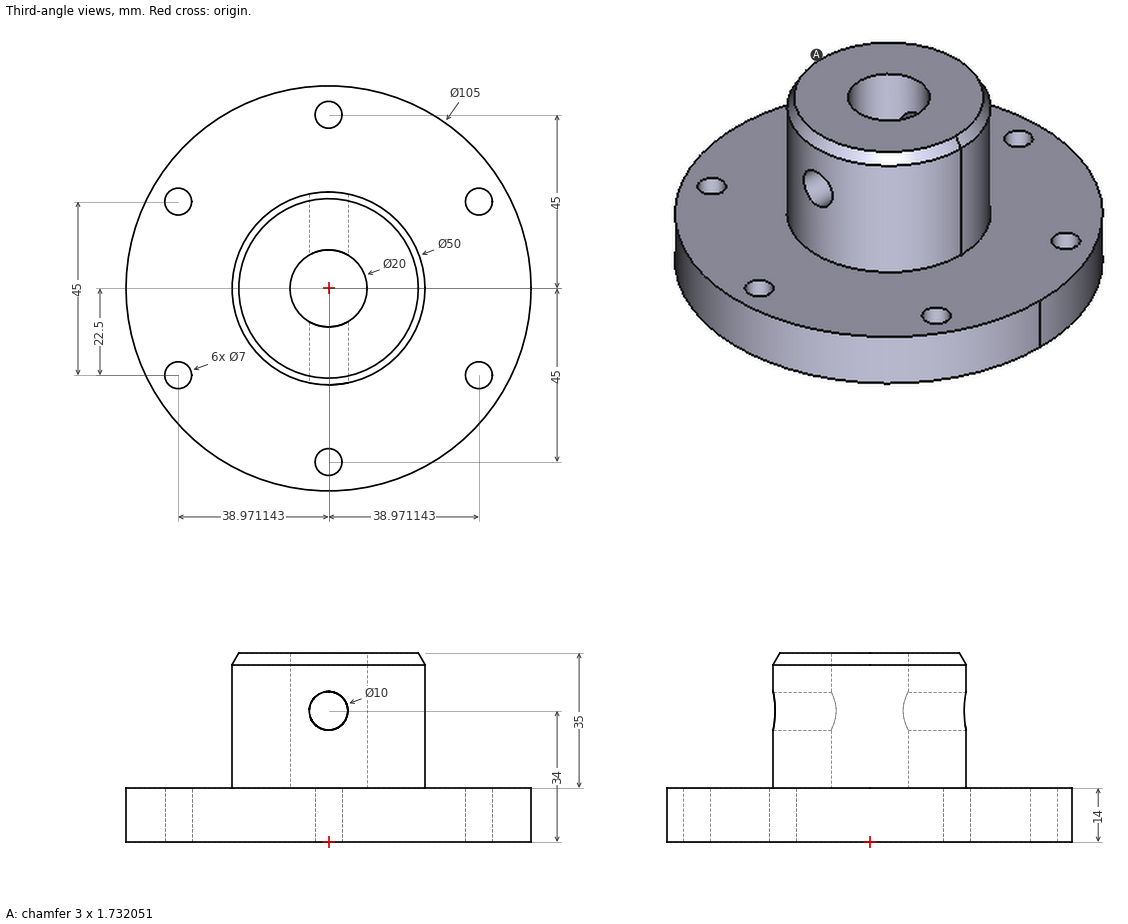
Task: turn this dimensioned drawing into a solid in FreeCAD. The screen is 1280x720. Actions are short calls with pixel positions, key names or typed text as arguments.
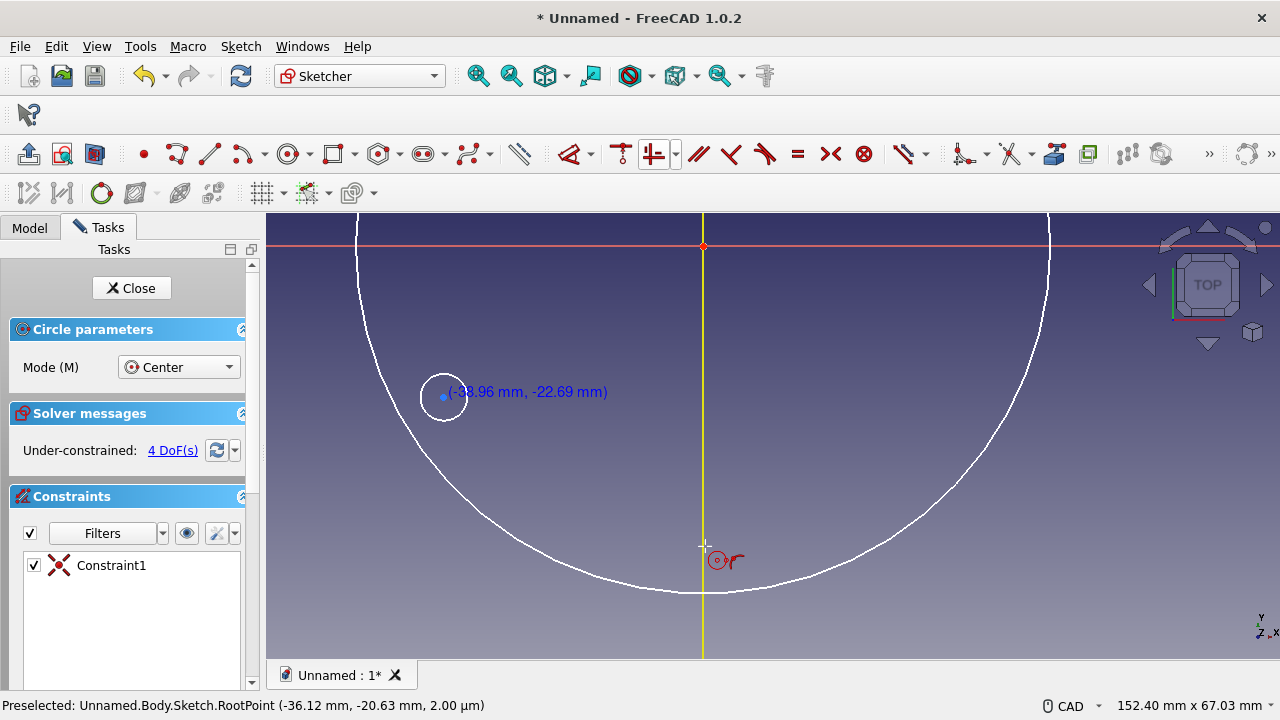
click(703, 546)
click(720, 529)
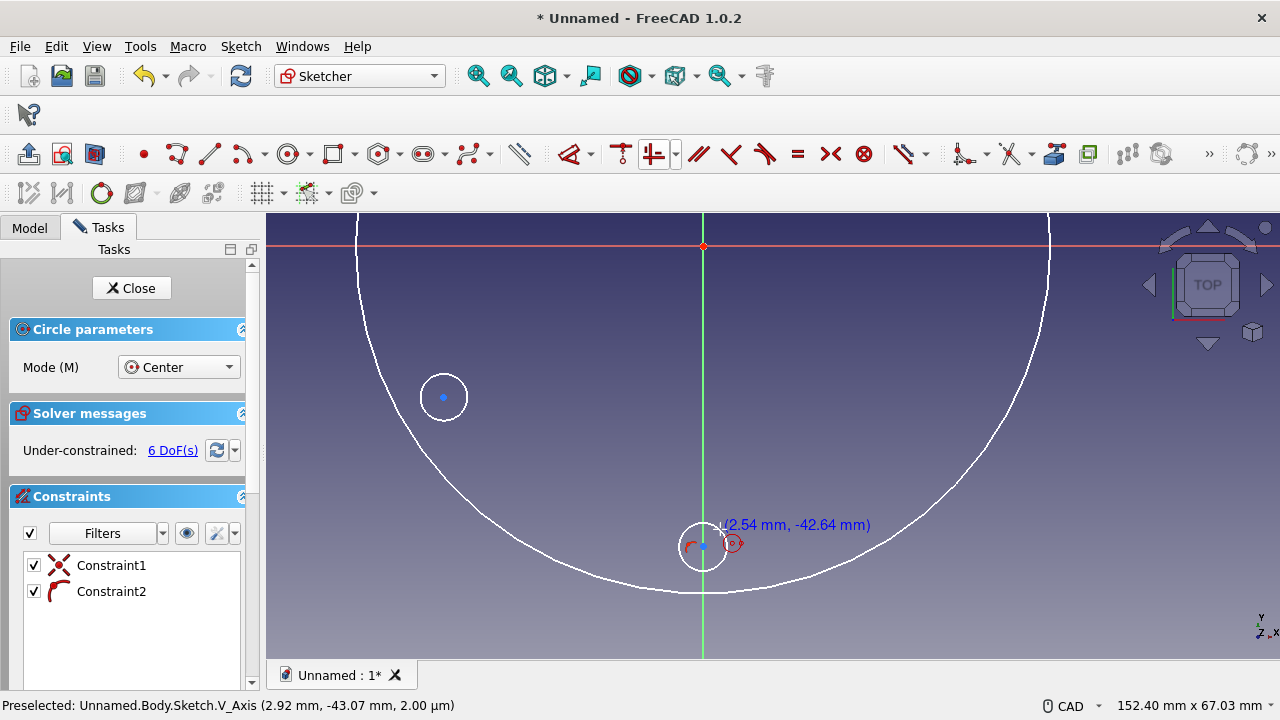
click(962, 396)
click(979, 380)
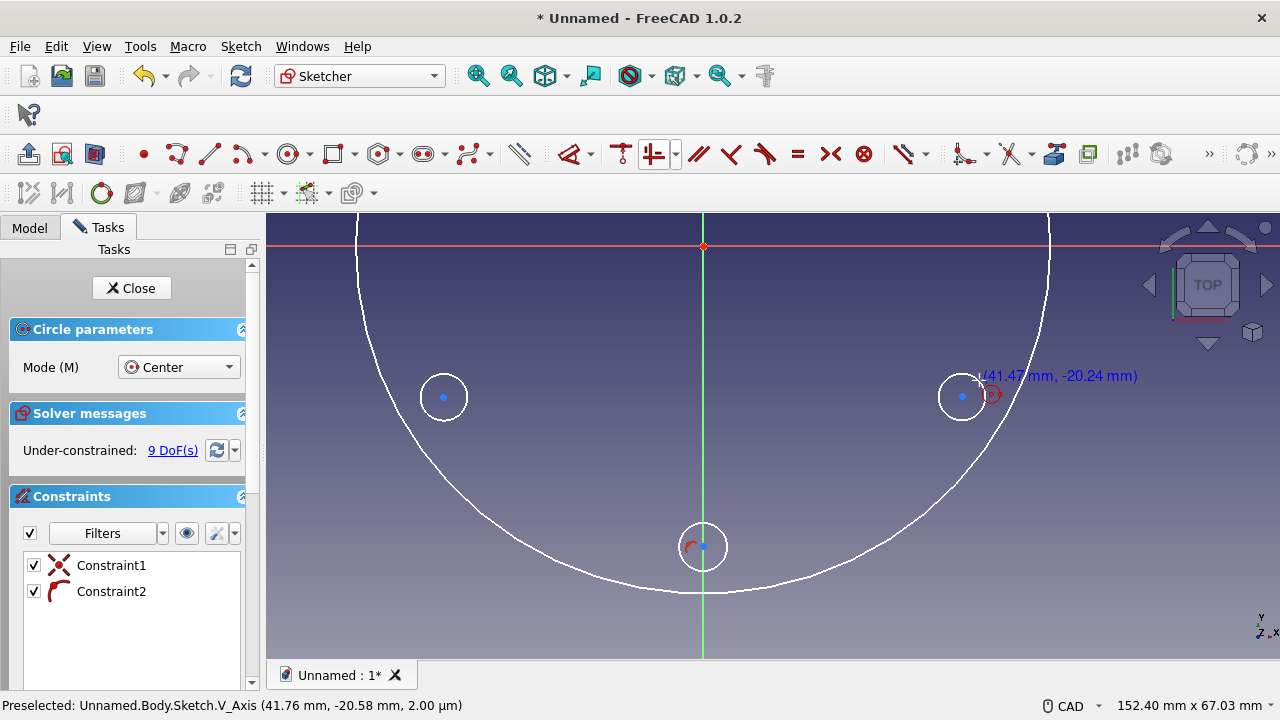
scroll(705, 546, down, 5)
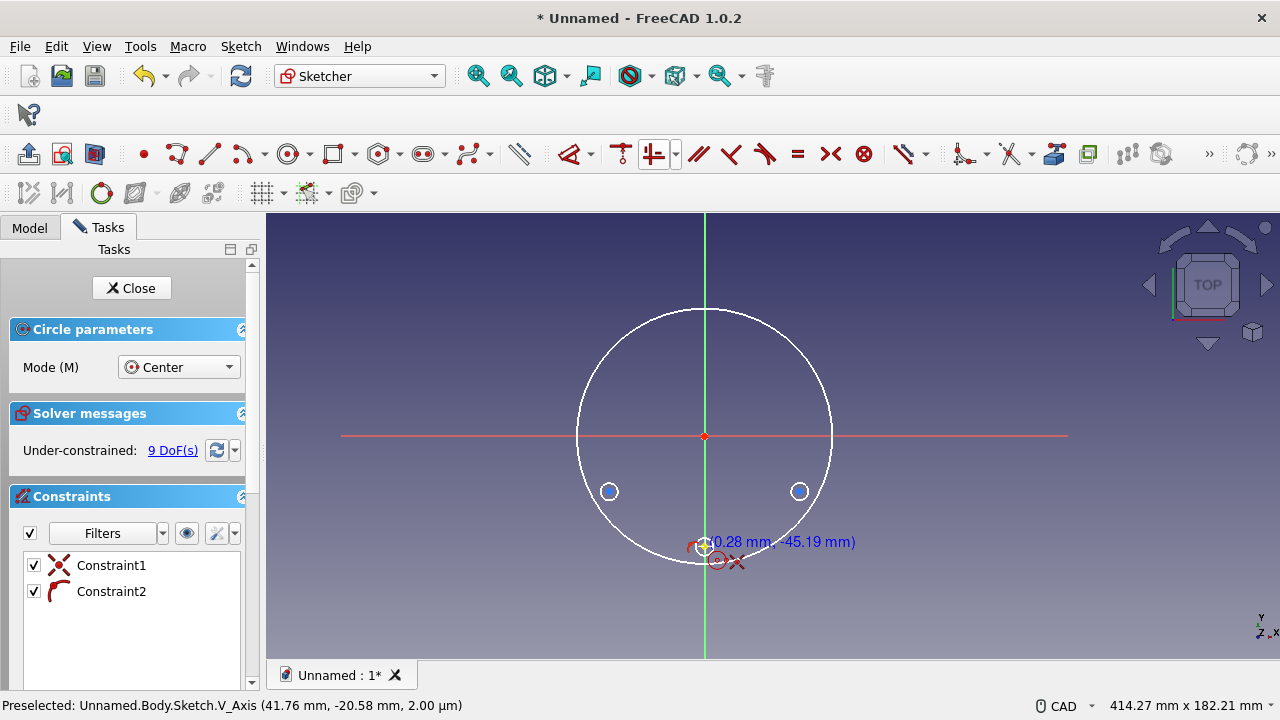
scroll(609, 381, up, 5)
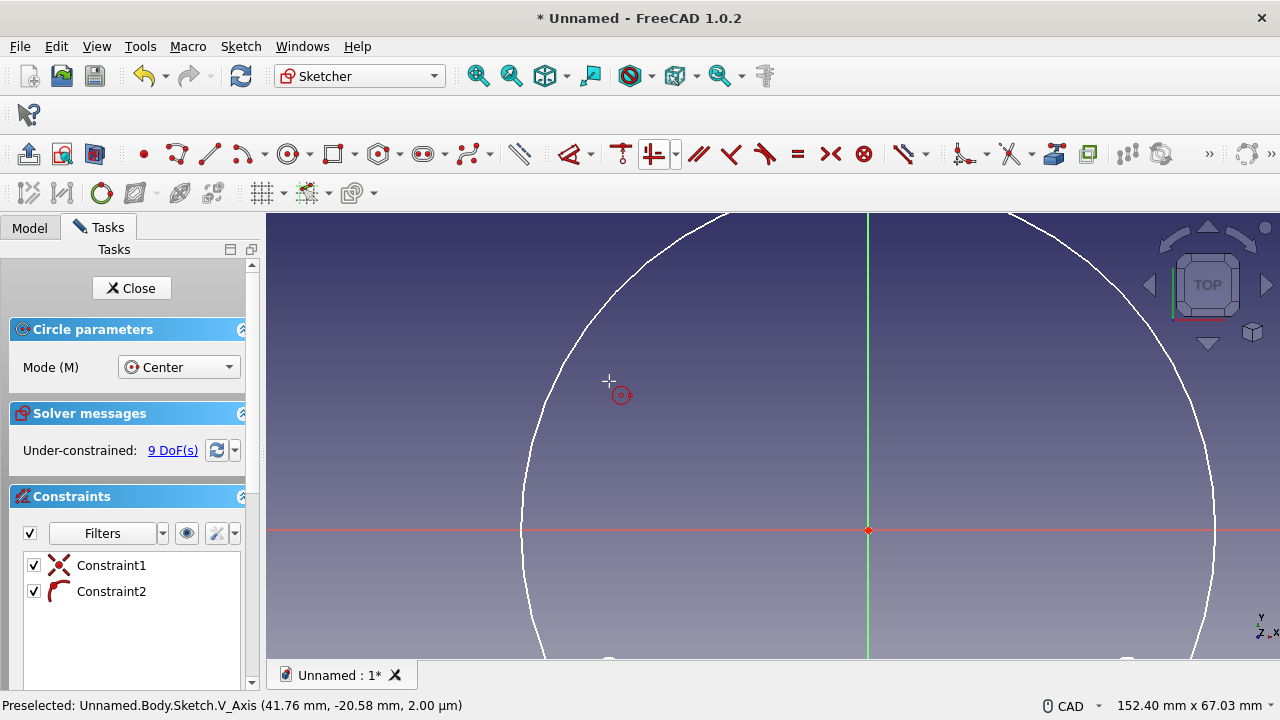
click(609, 381)
click(625, 364)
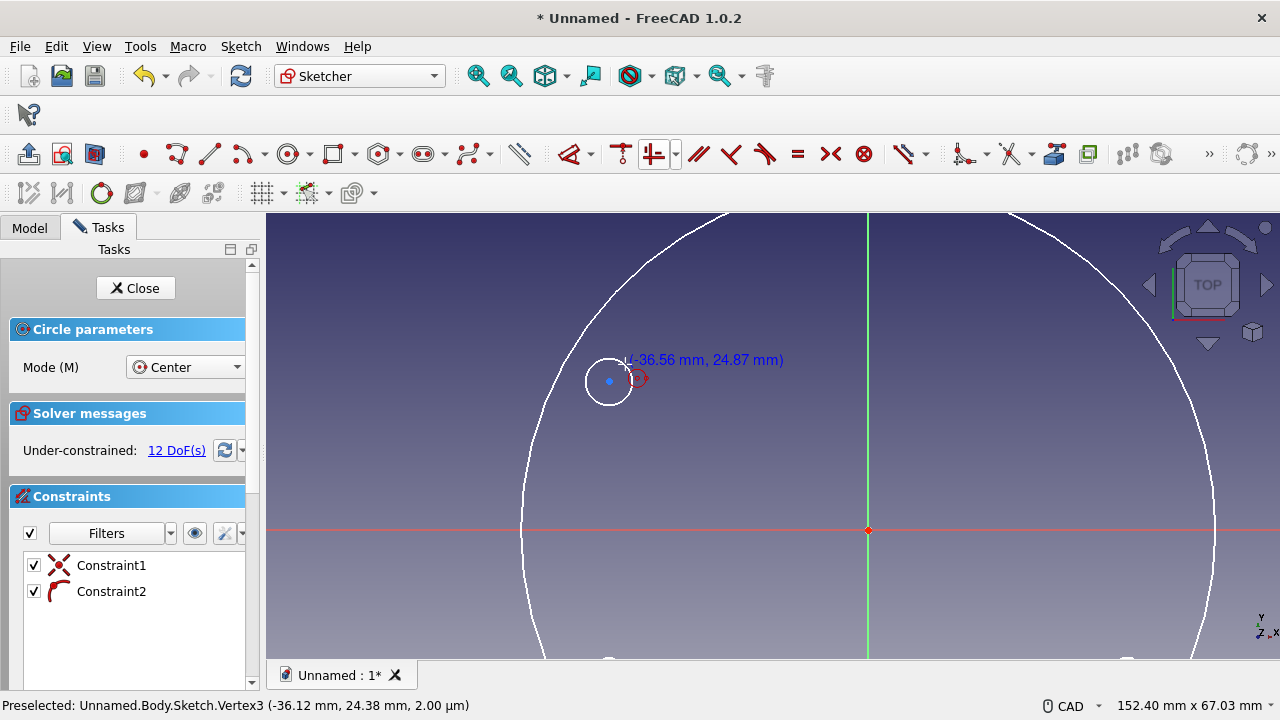
scroll(609, 381, down, 5)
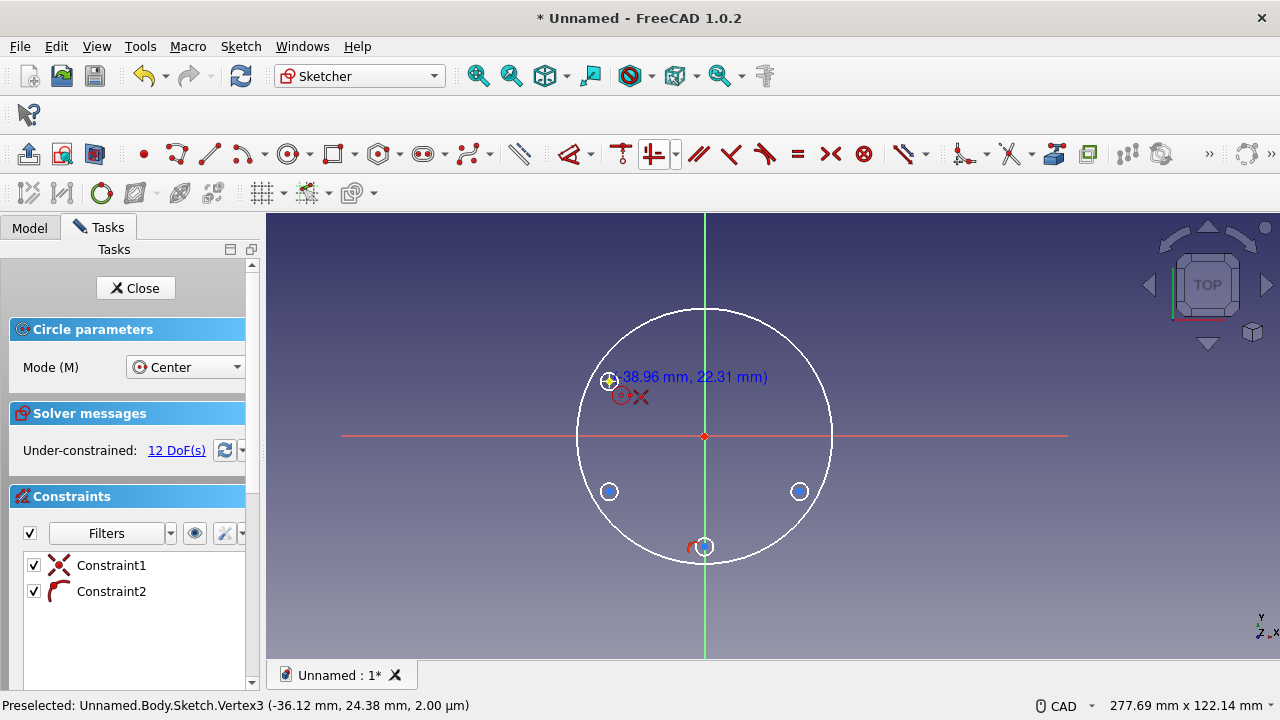
scroll(800, 381, up, 5)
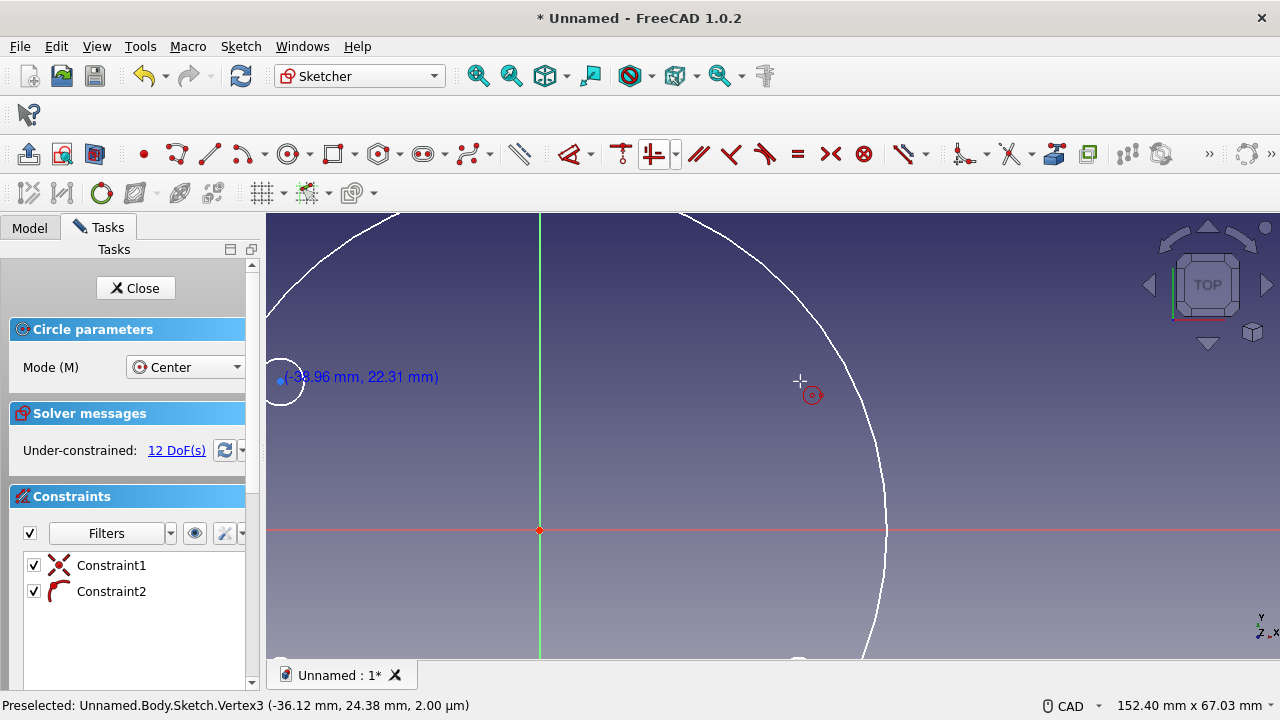
click(799, 381)
click(815, 364)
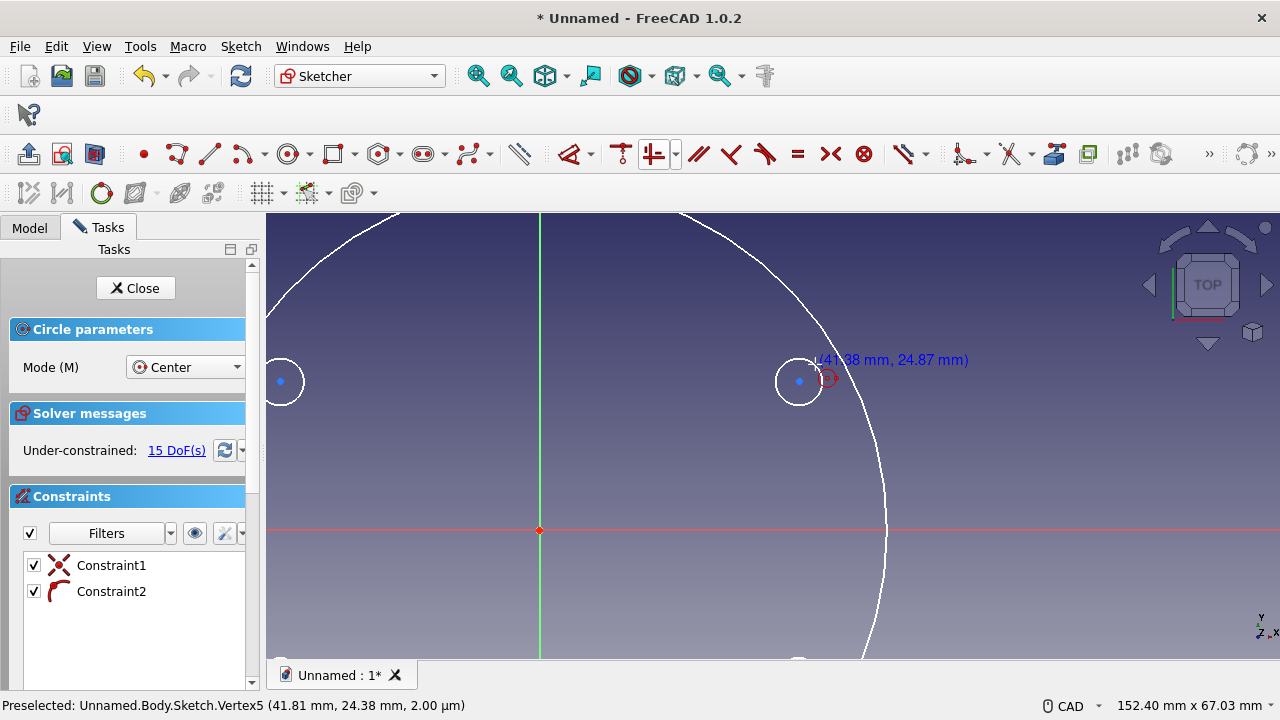
scroll(800, 381, down, 5)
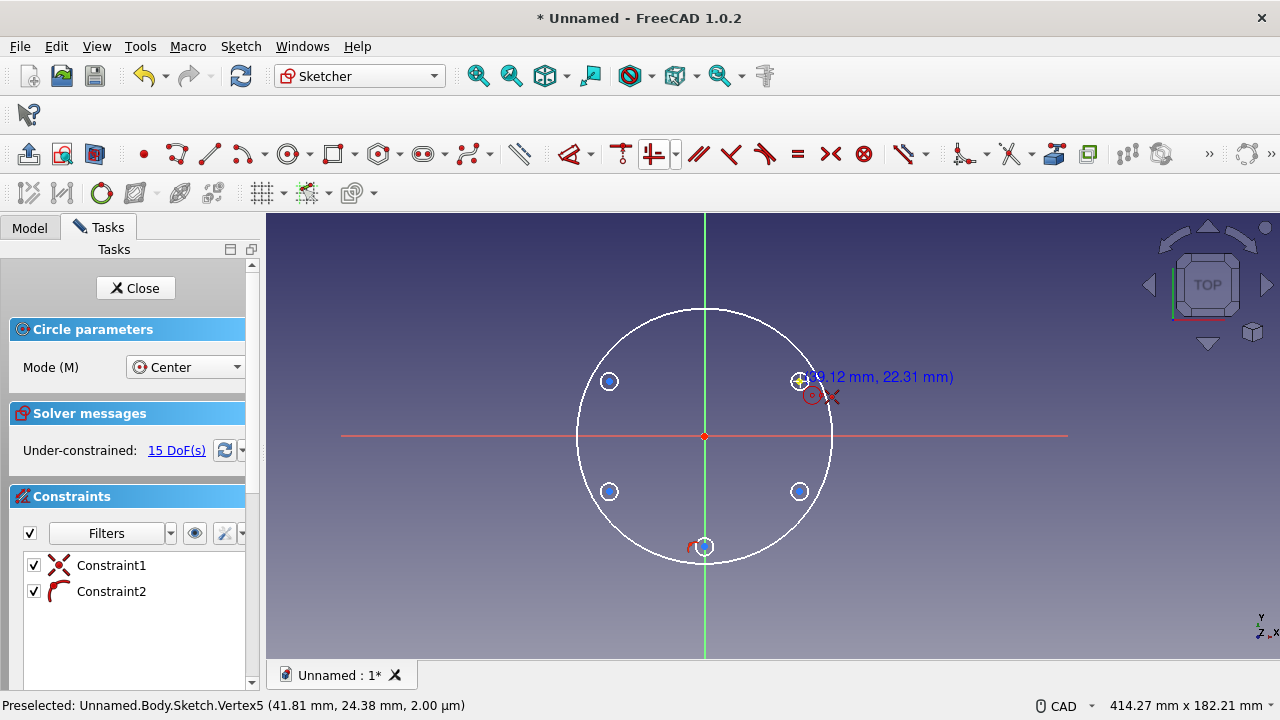
scroll(705, 326, up, 5)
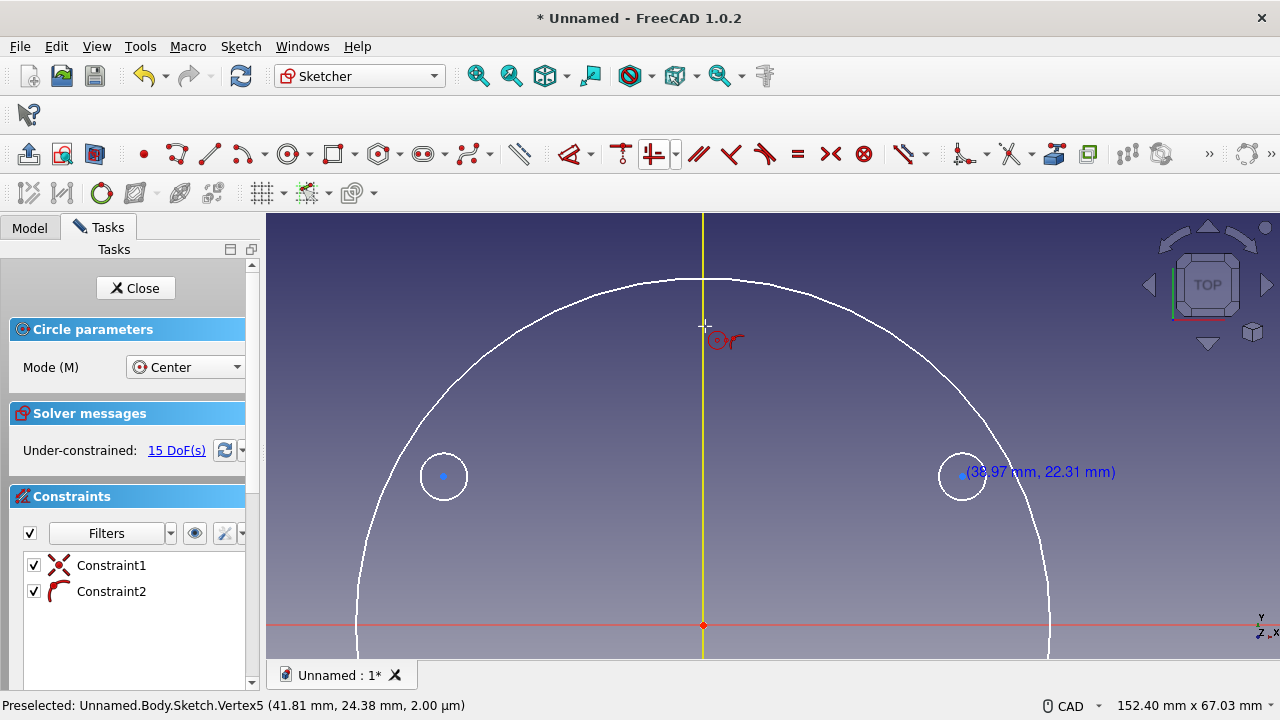
click(703, 326)
click(720, 309)
key(Escape)